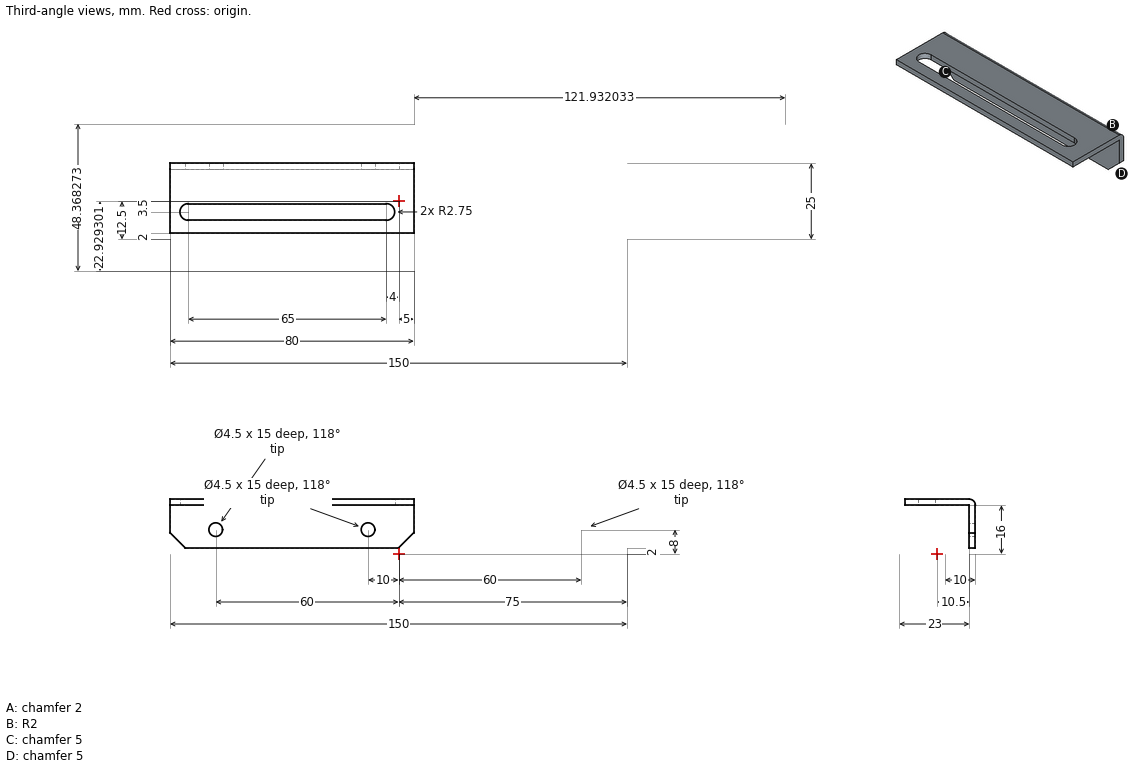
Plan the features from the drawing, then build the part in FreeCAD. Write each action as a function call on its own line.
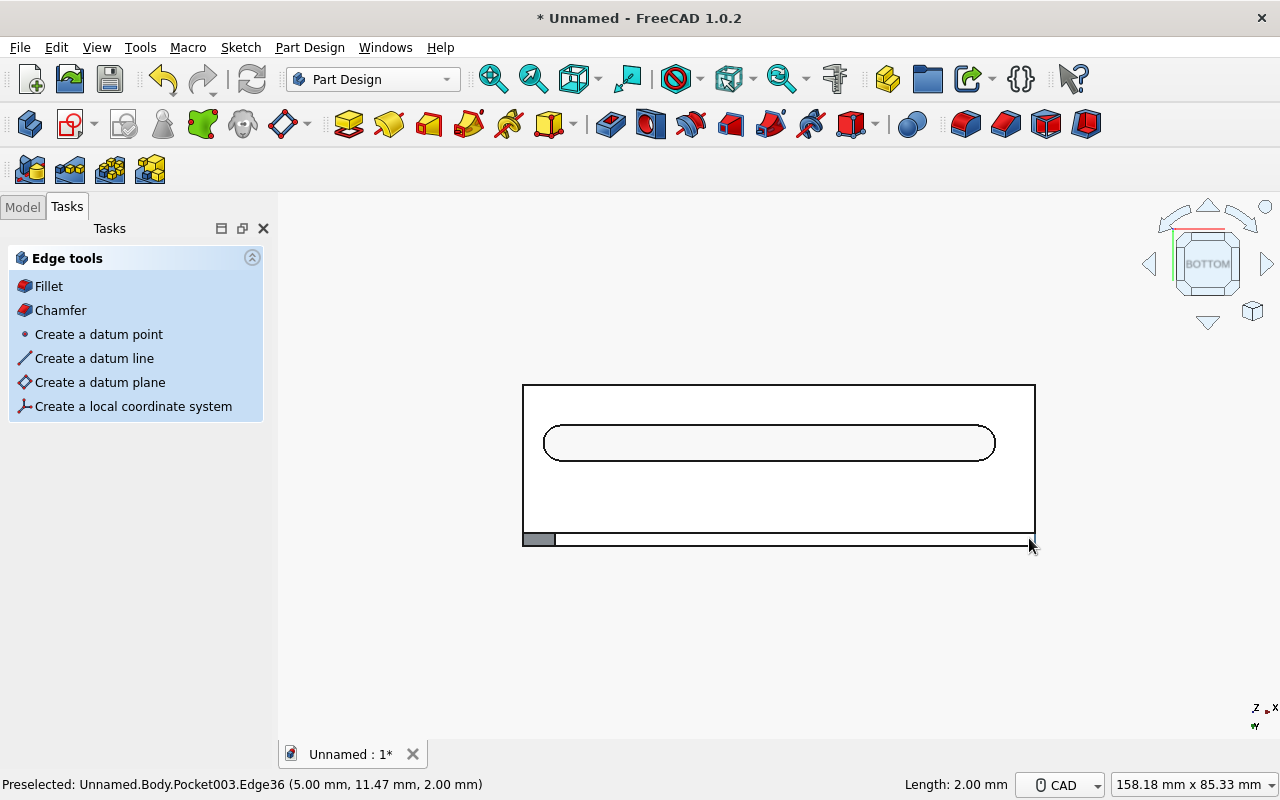
click(1006, 124)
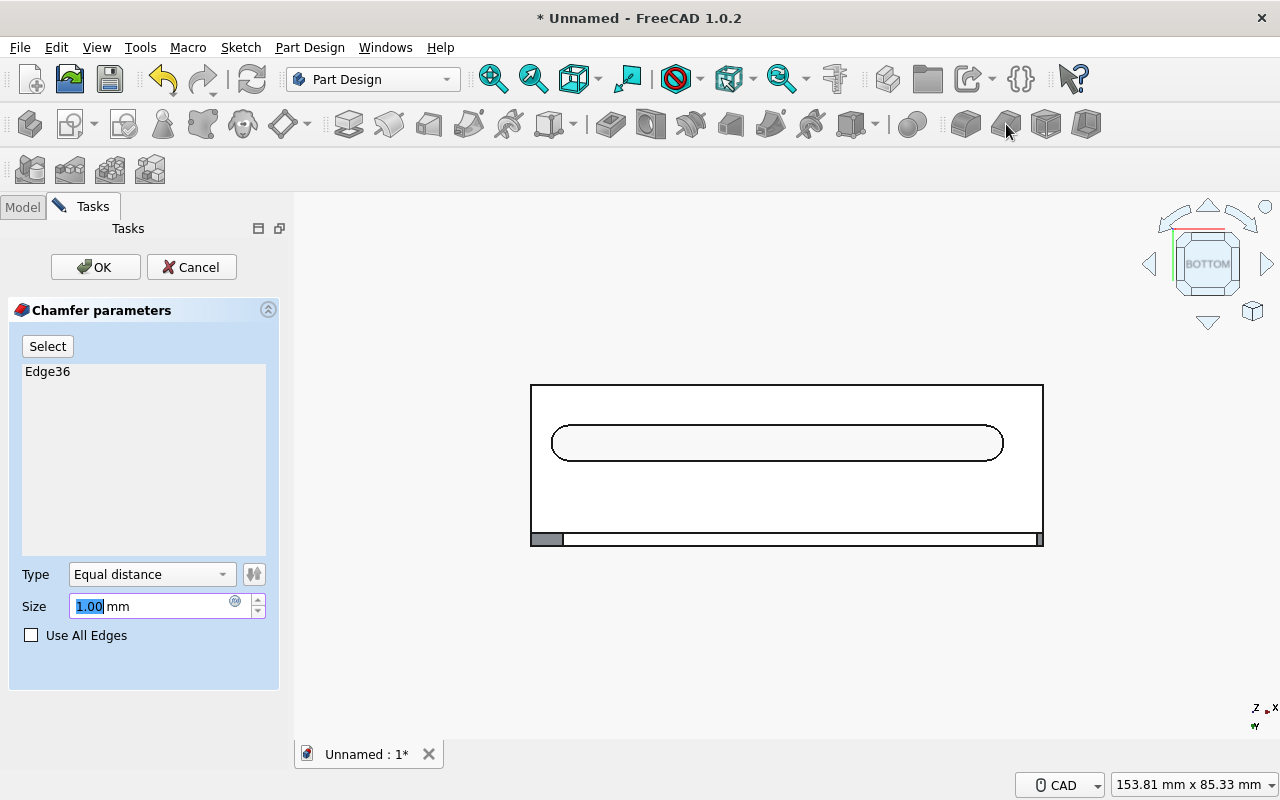
text(5)
key(Tab)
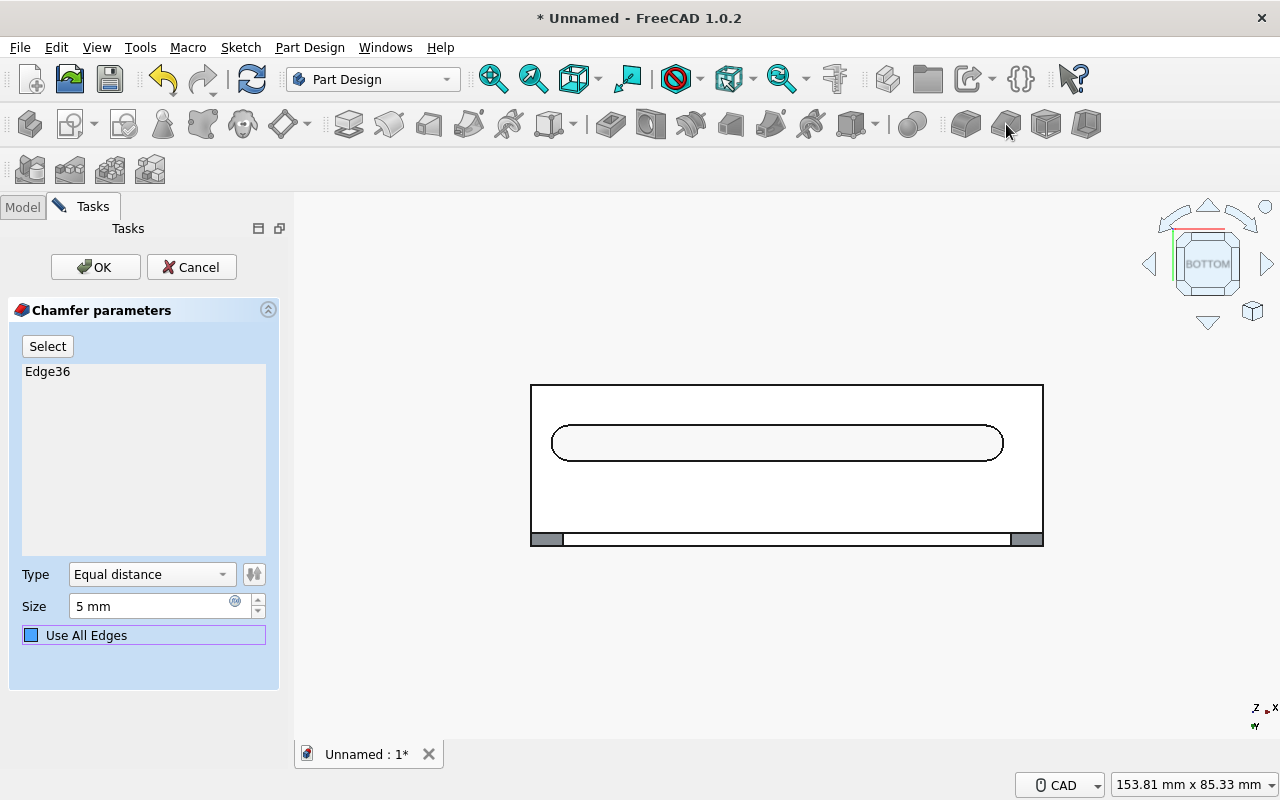
click(96, 267)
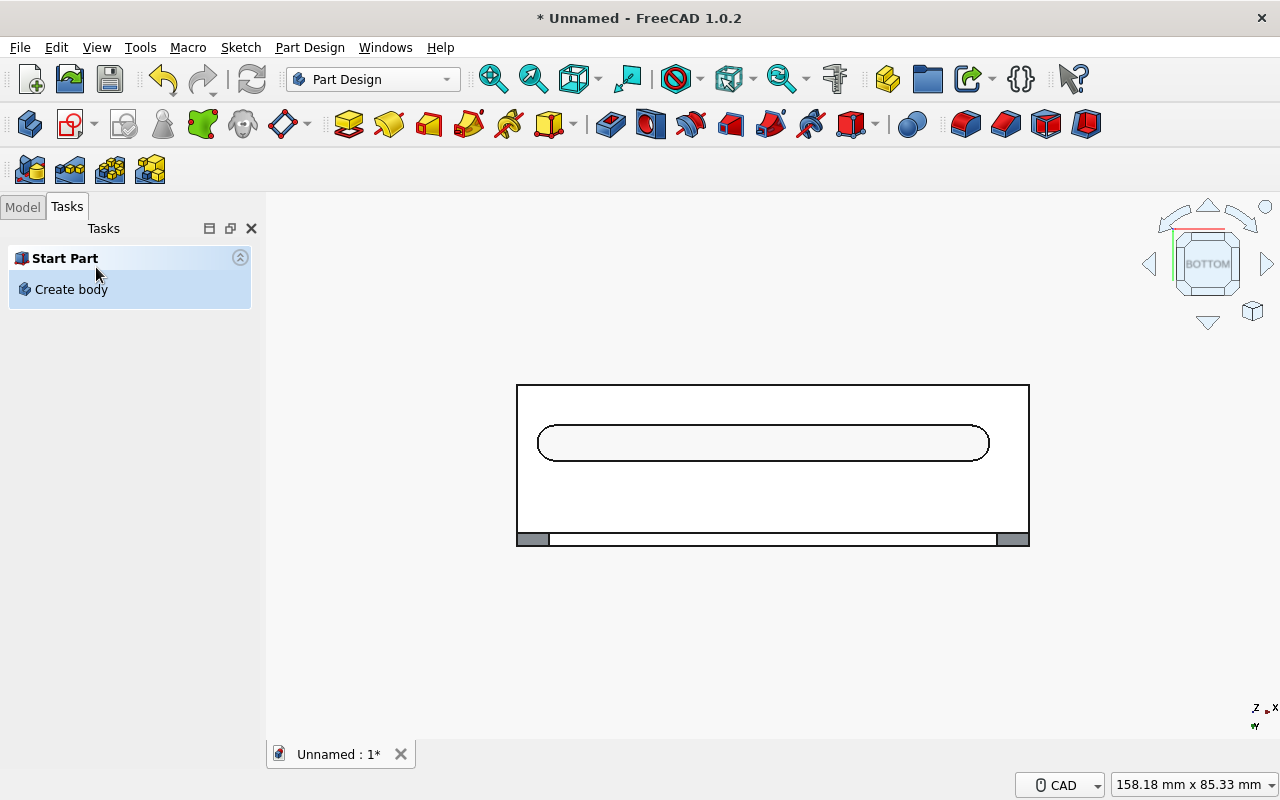
click(993, 500)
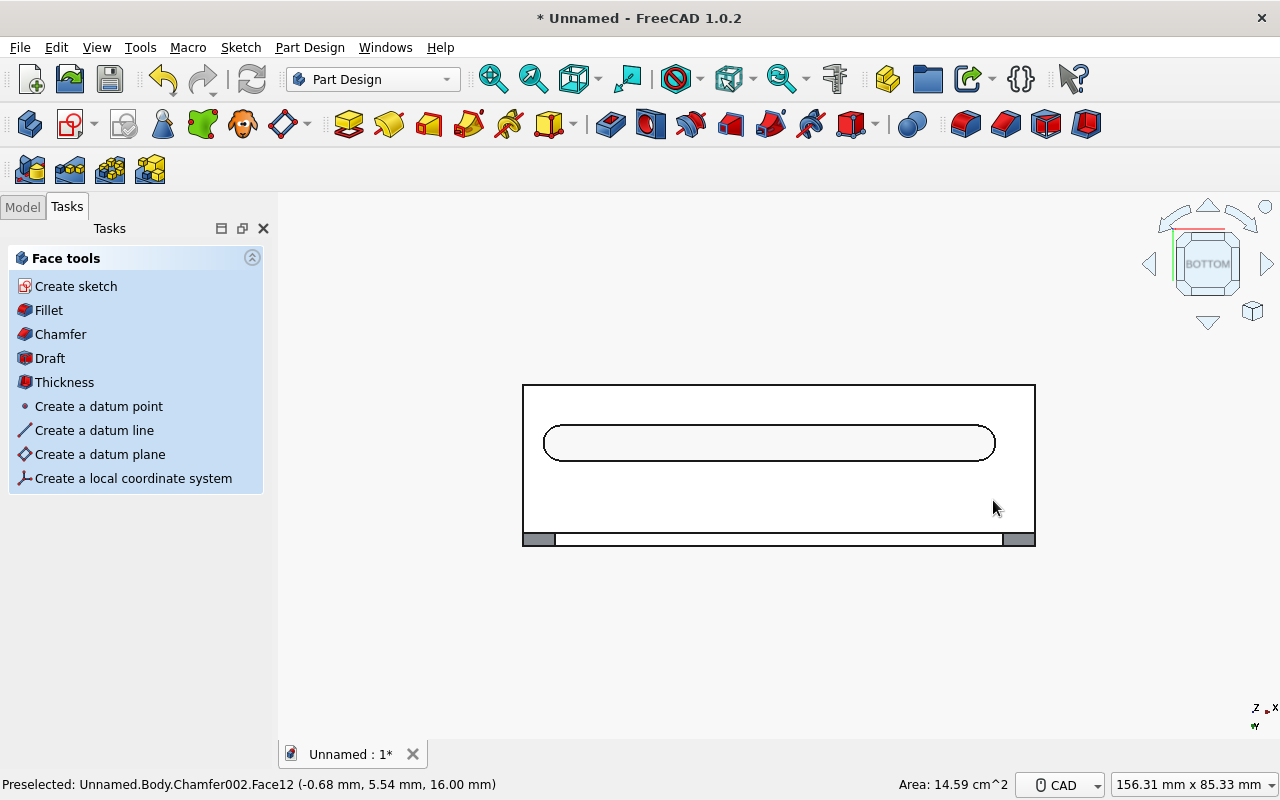
click(70, 124)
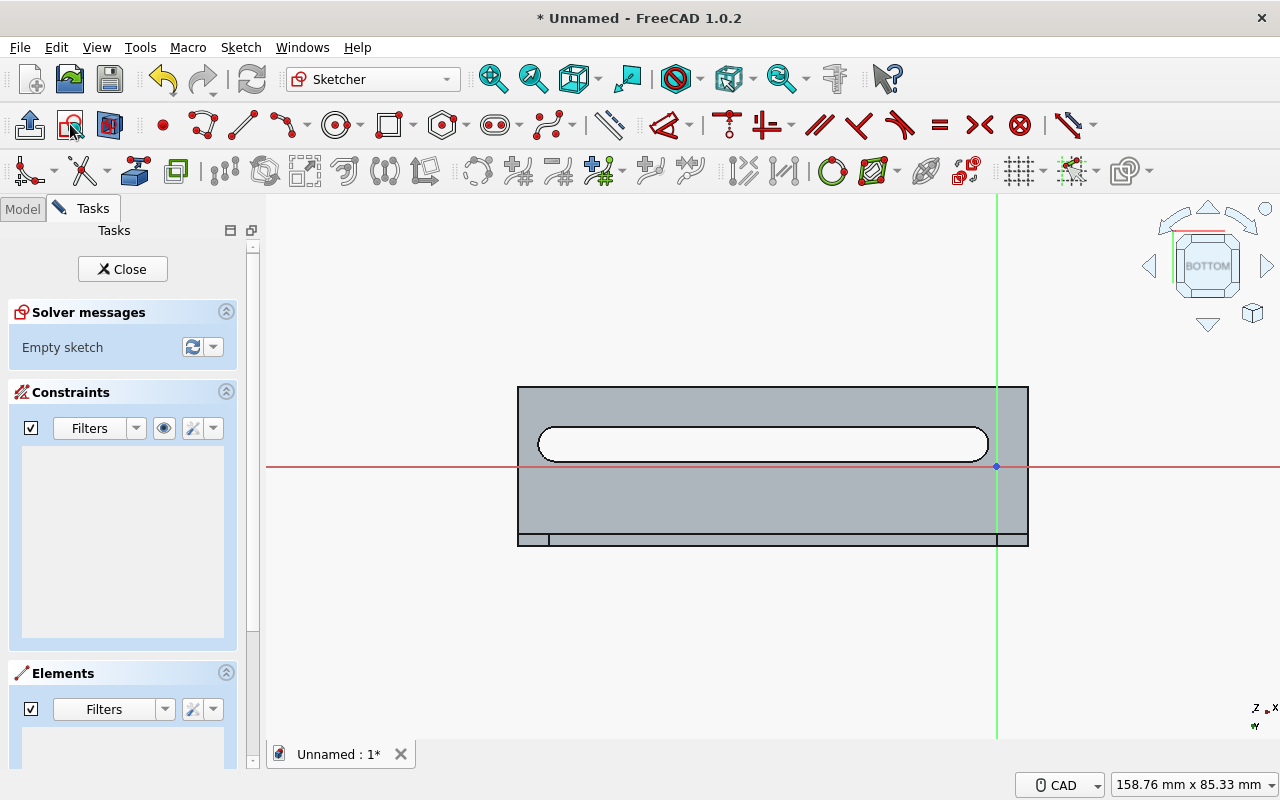
click(110, 126)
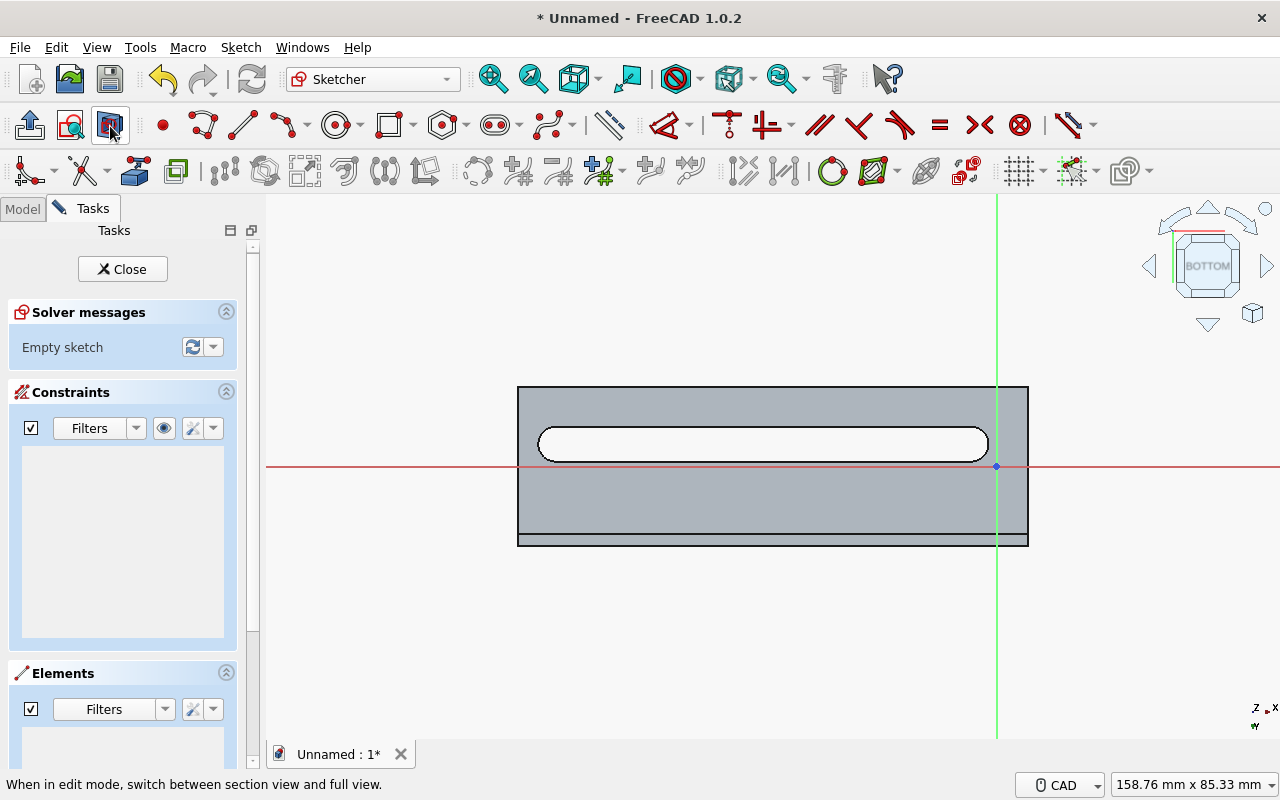
click(390, 126)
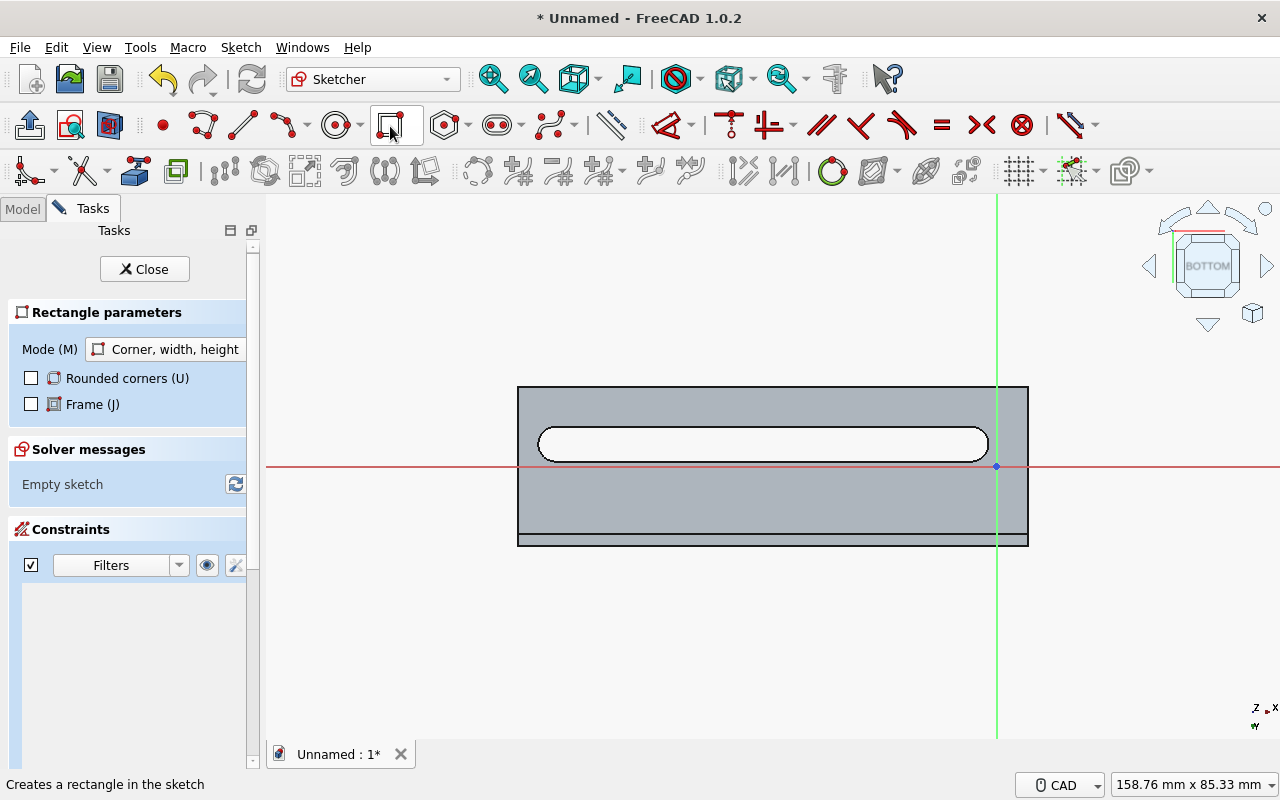
scroll(518, 387, up, 2)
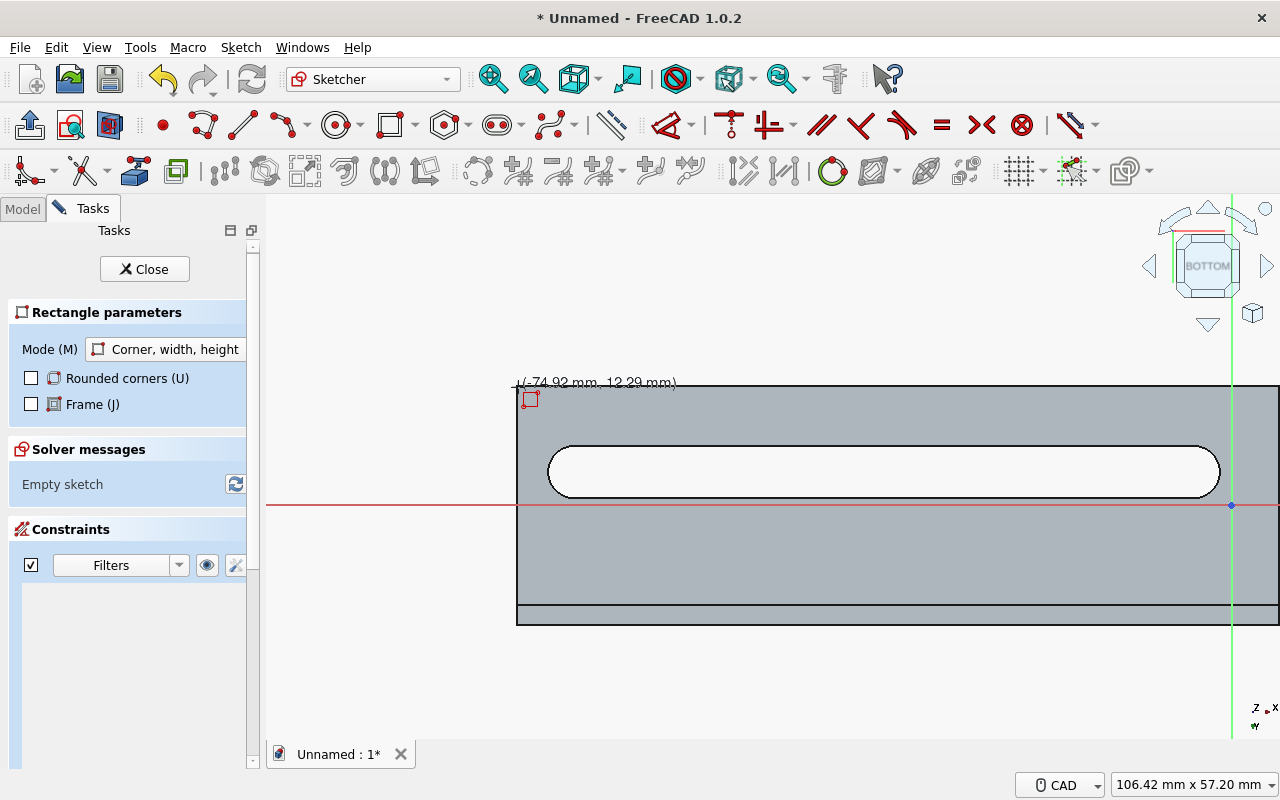
click(517, 386)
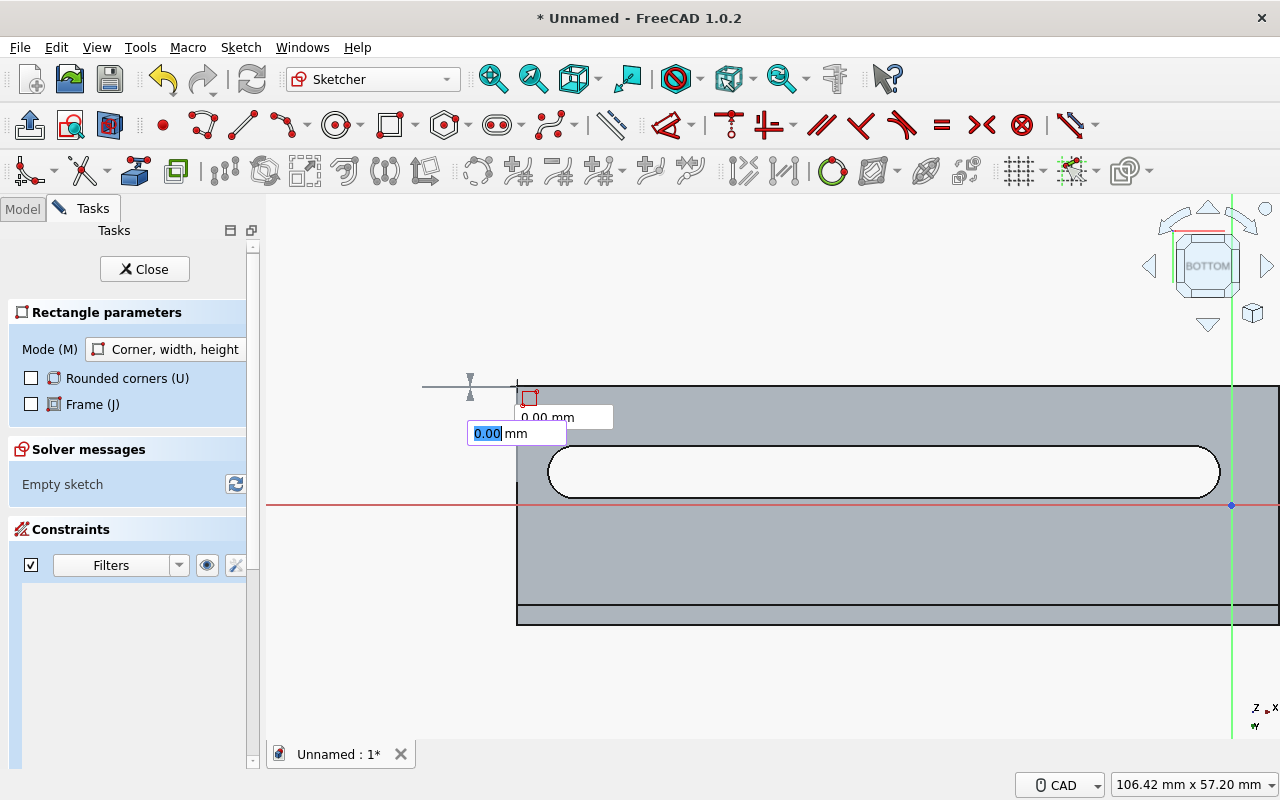
scroll(310, 508, down, 2)